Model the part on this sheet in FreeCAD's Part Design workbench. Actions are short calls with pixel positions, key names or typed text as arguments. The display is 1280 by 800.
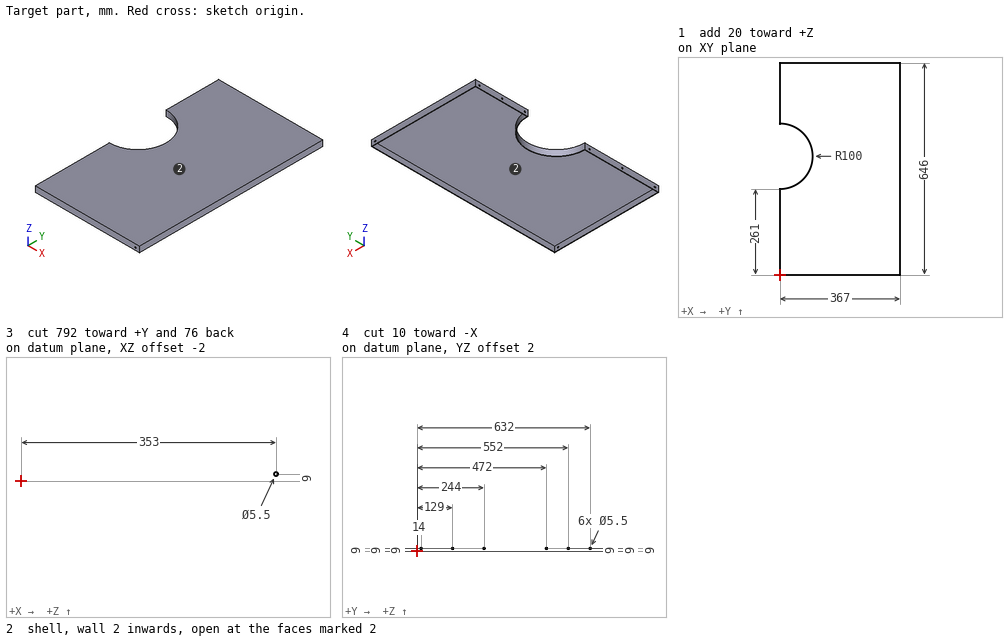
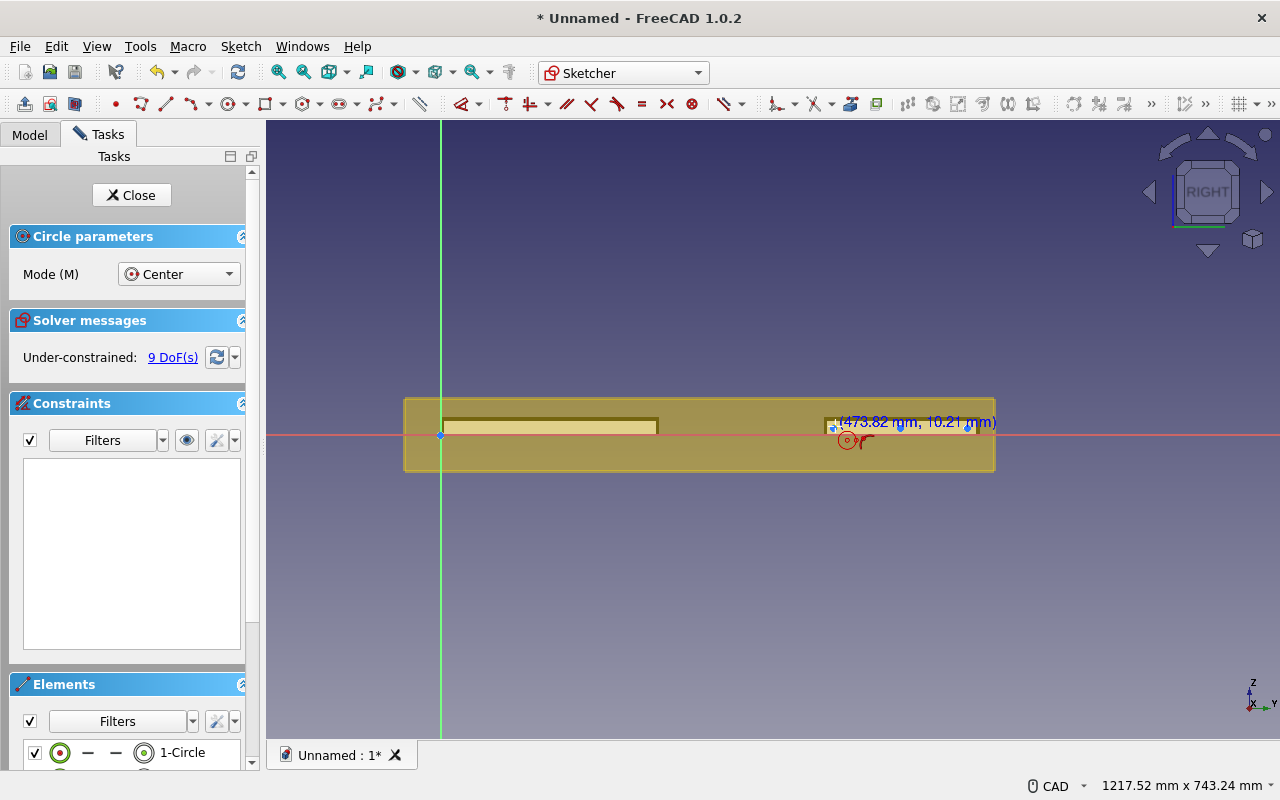
scroll(453, 428, up, 12)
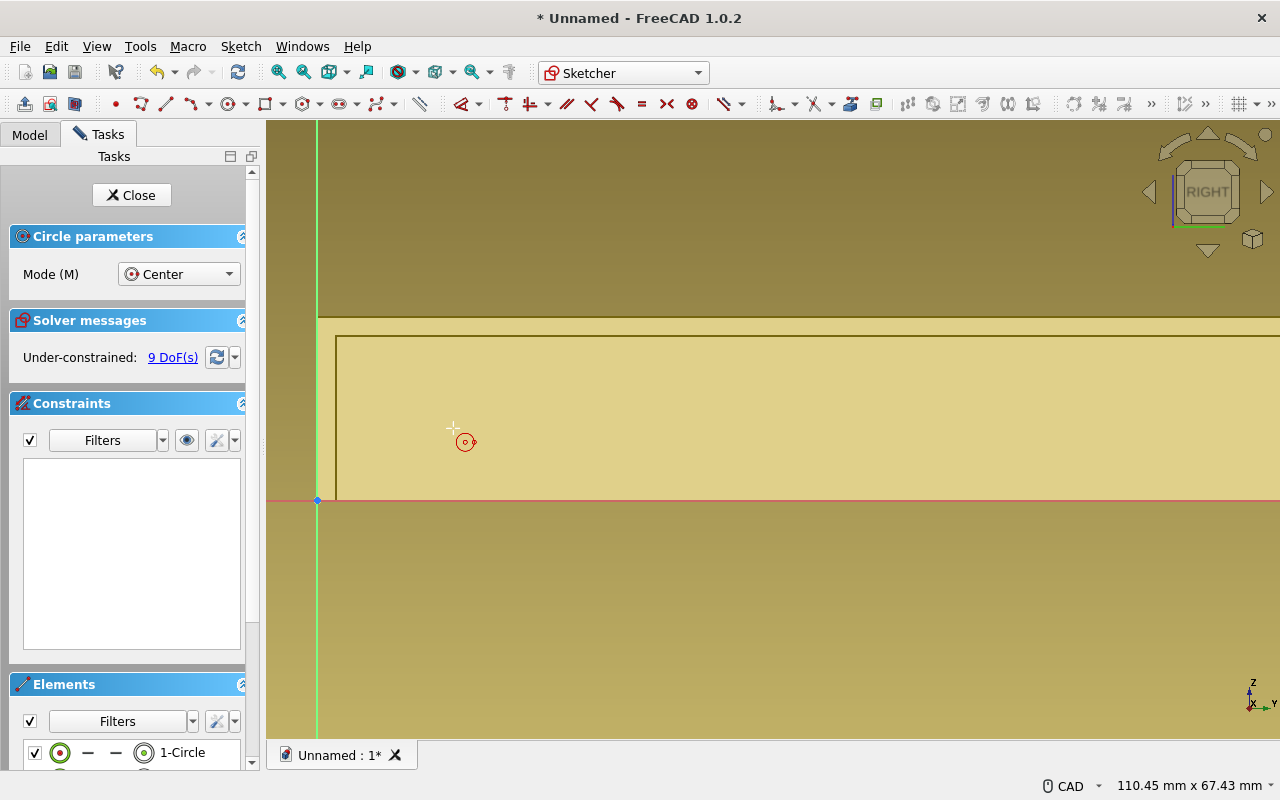
scroll(452, 428, down, 12)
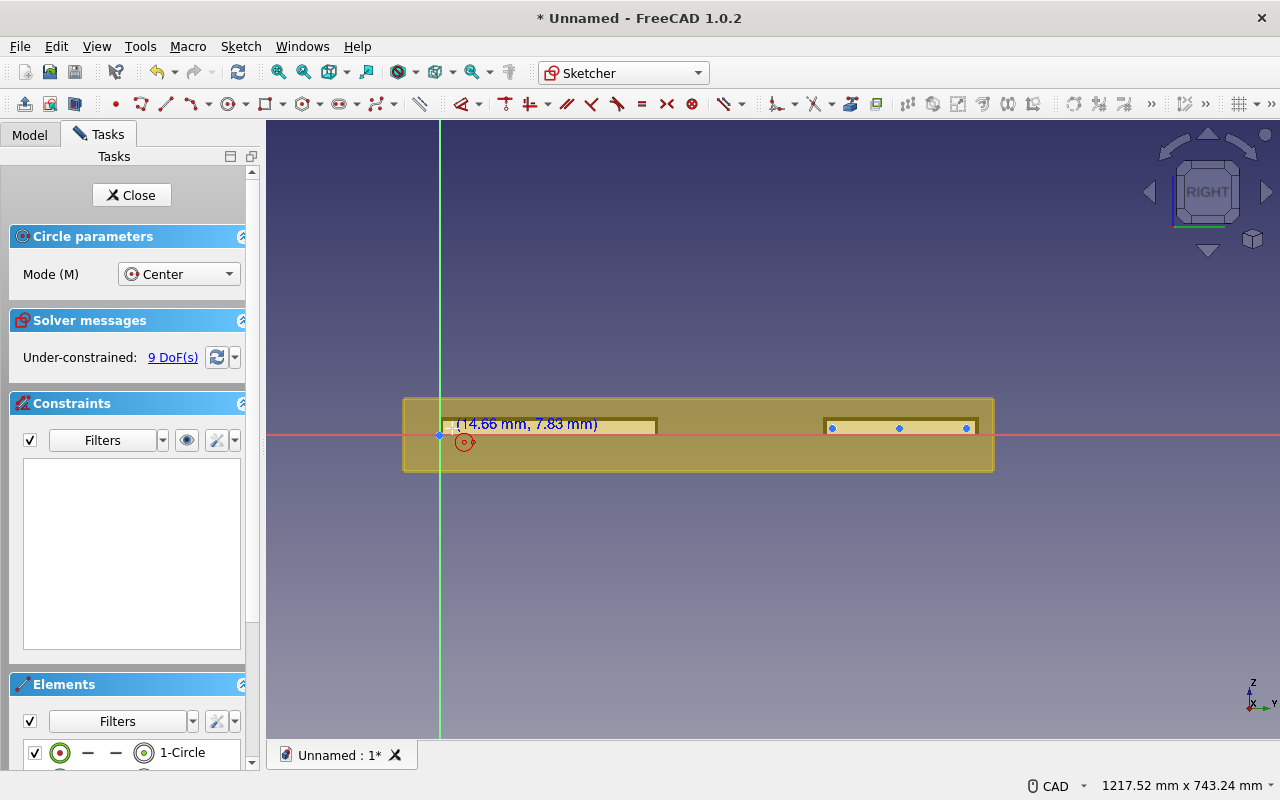
scroll(452, 428, up, 4)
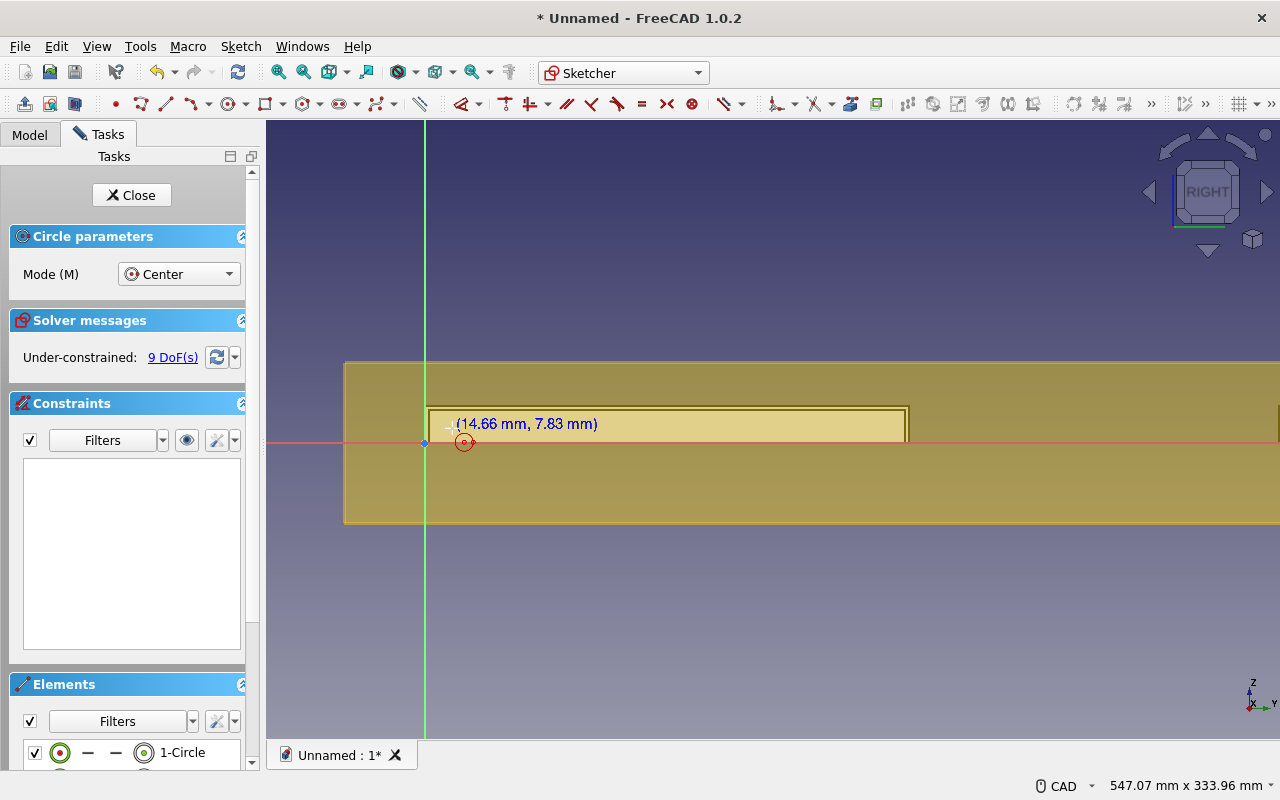
click(451, 426)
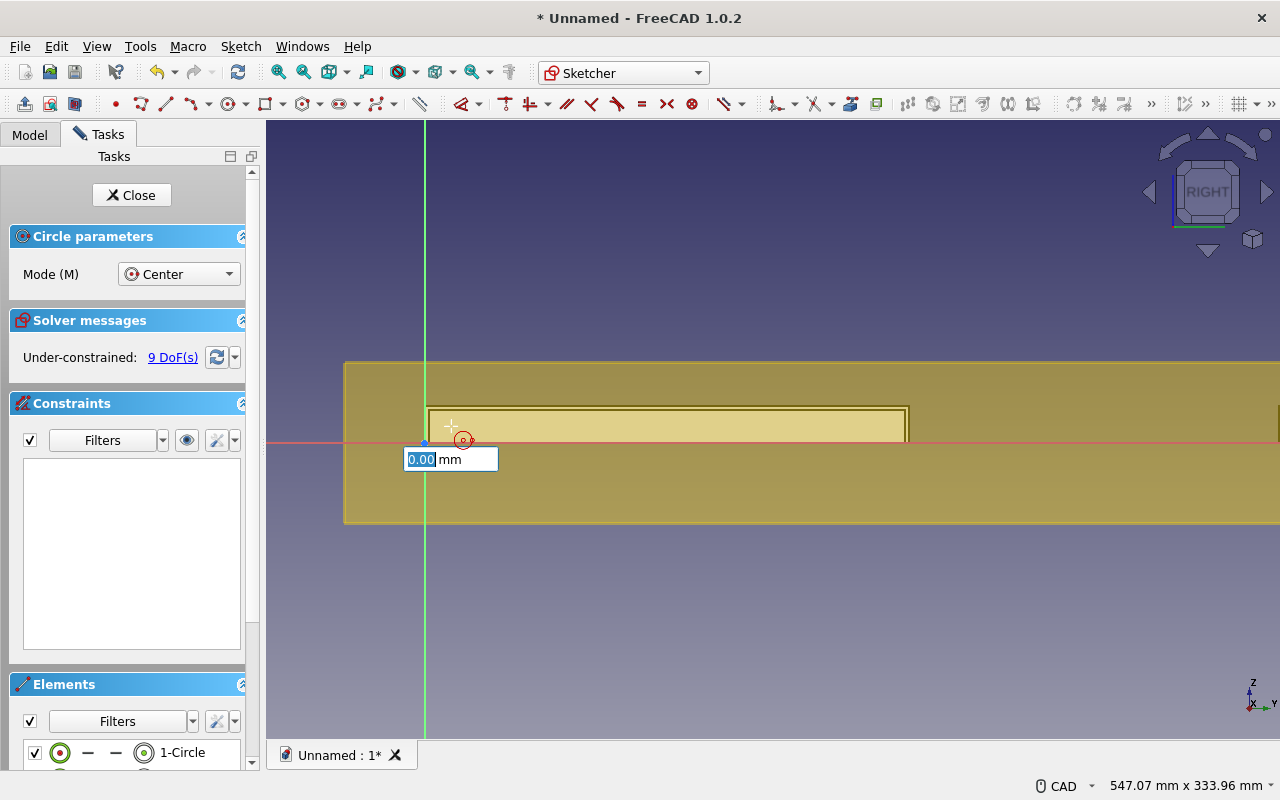
scroll(455, 423, up, 6)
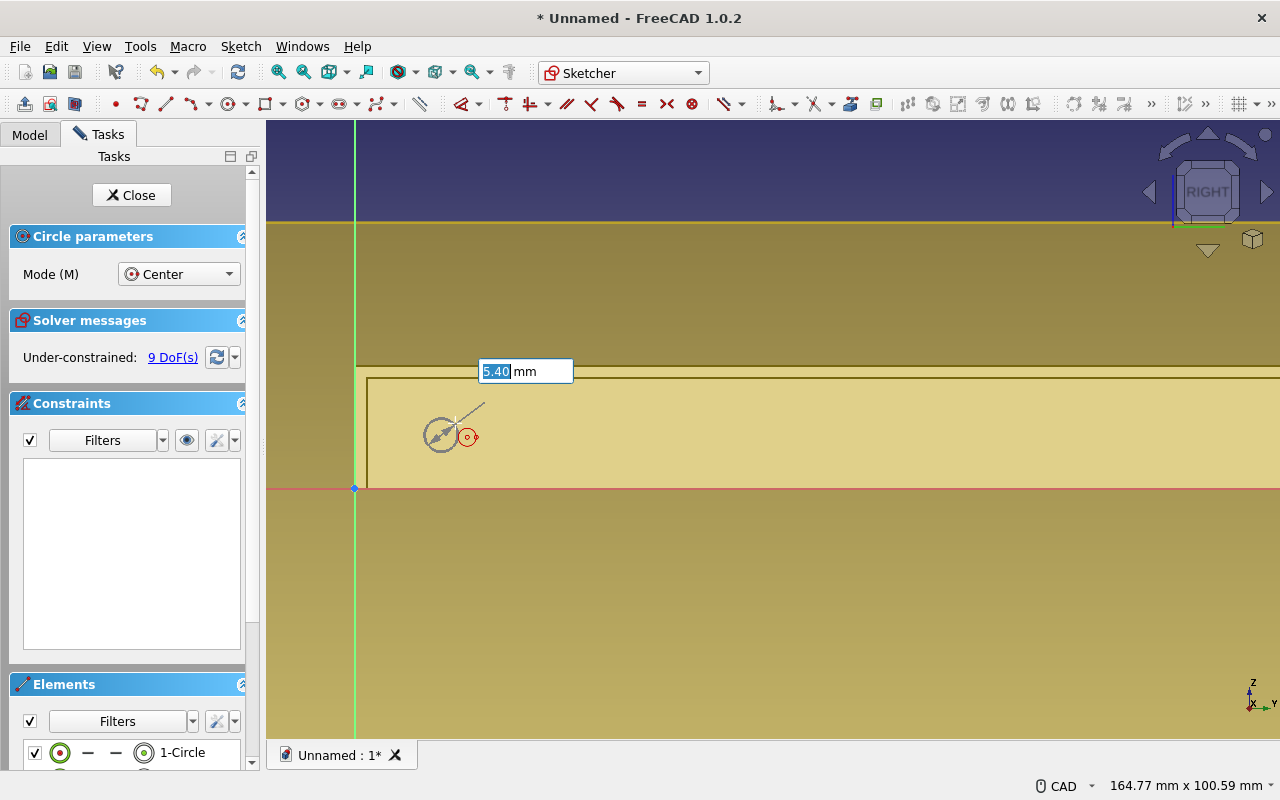
click(453, 421)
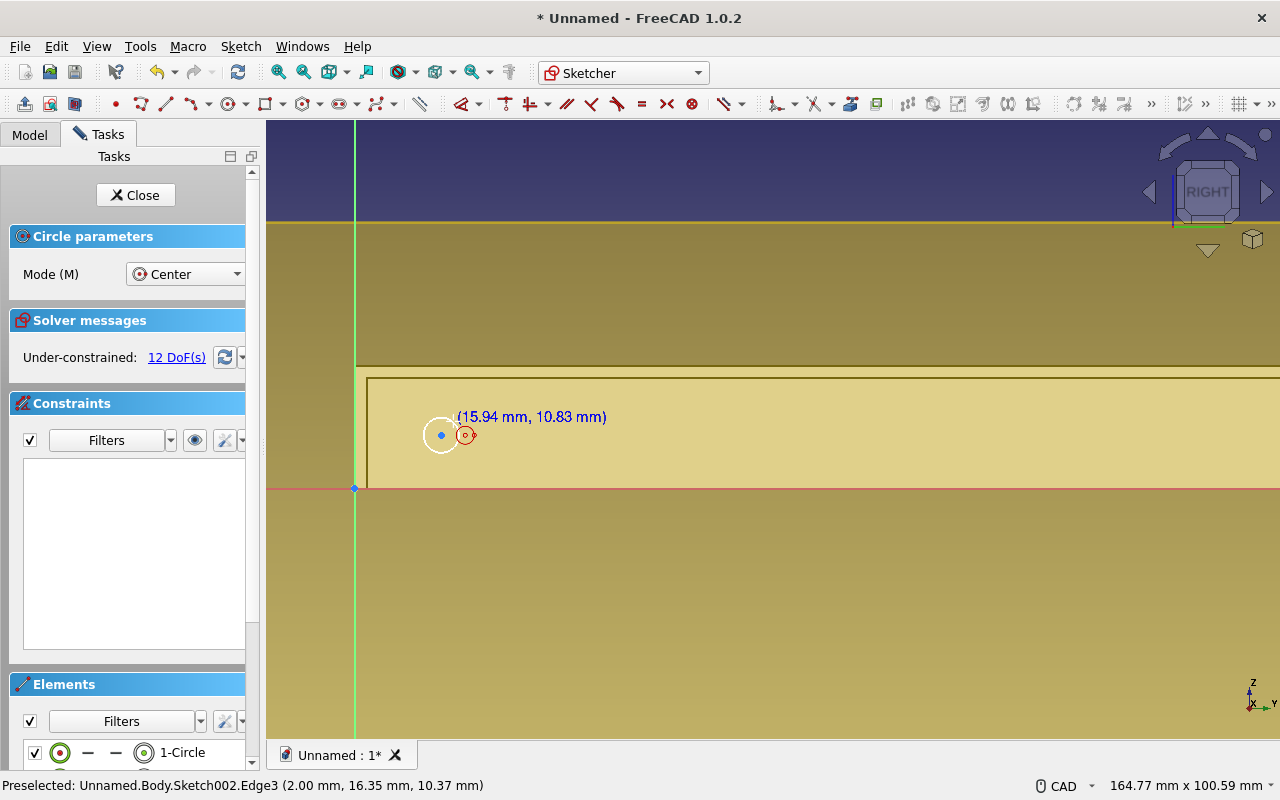
scroll(454, 426, down, 10)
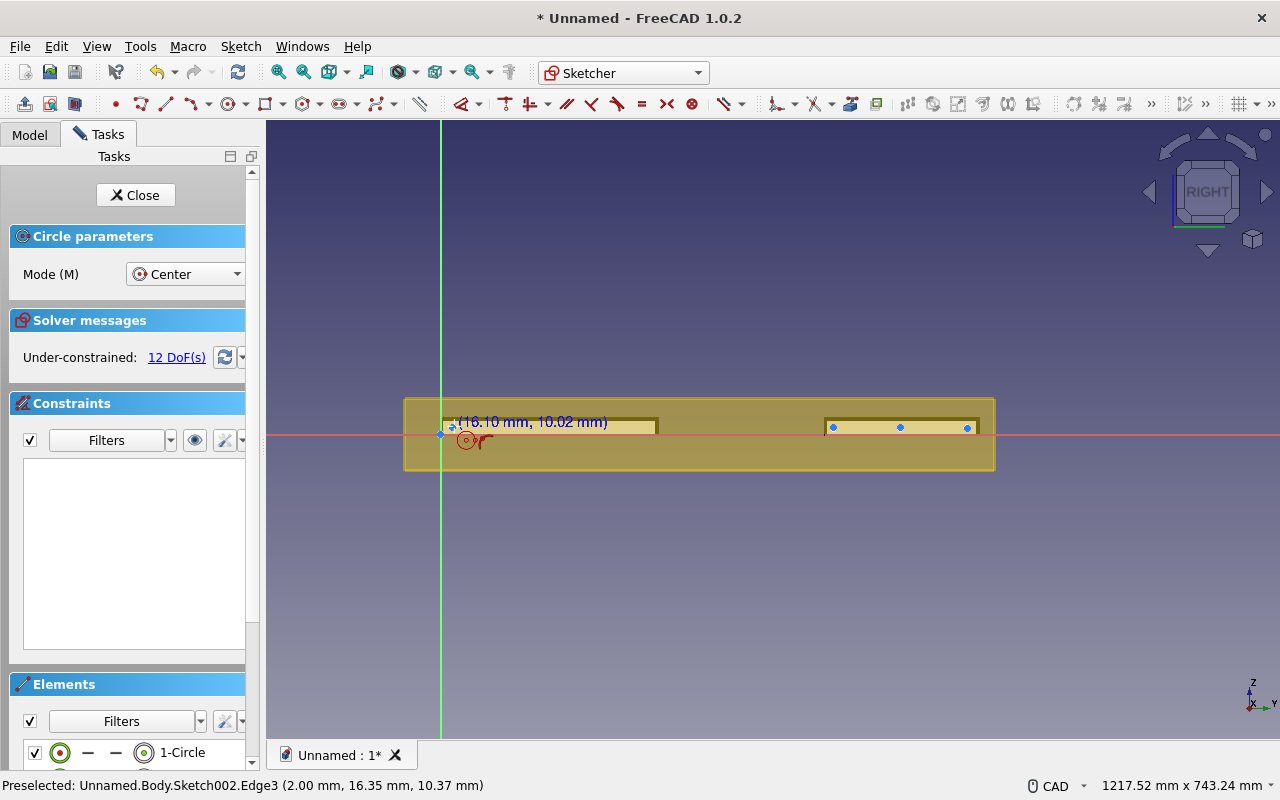
scroll(548, 427, up, 12)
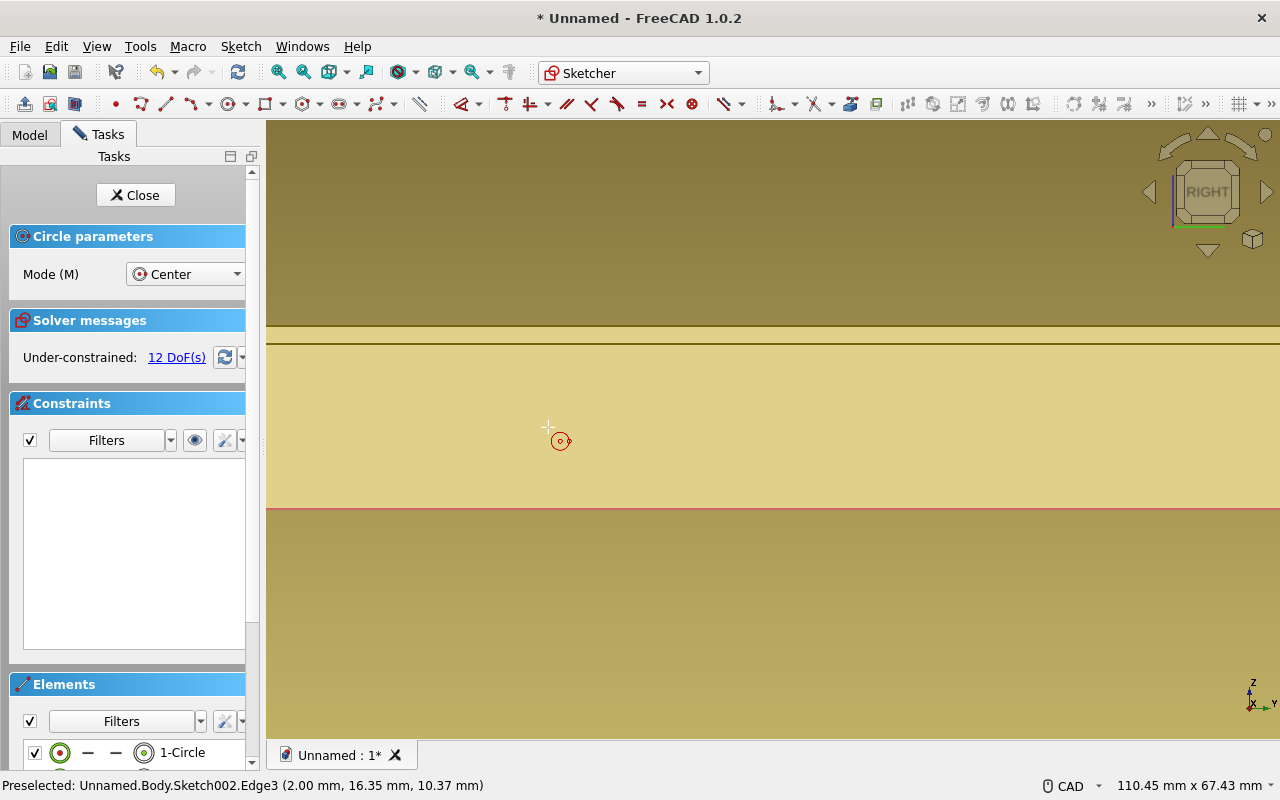
scroll(548, 427, down, 12)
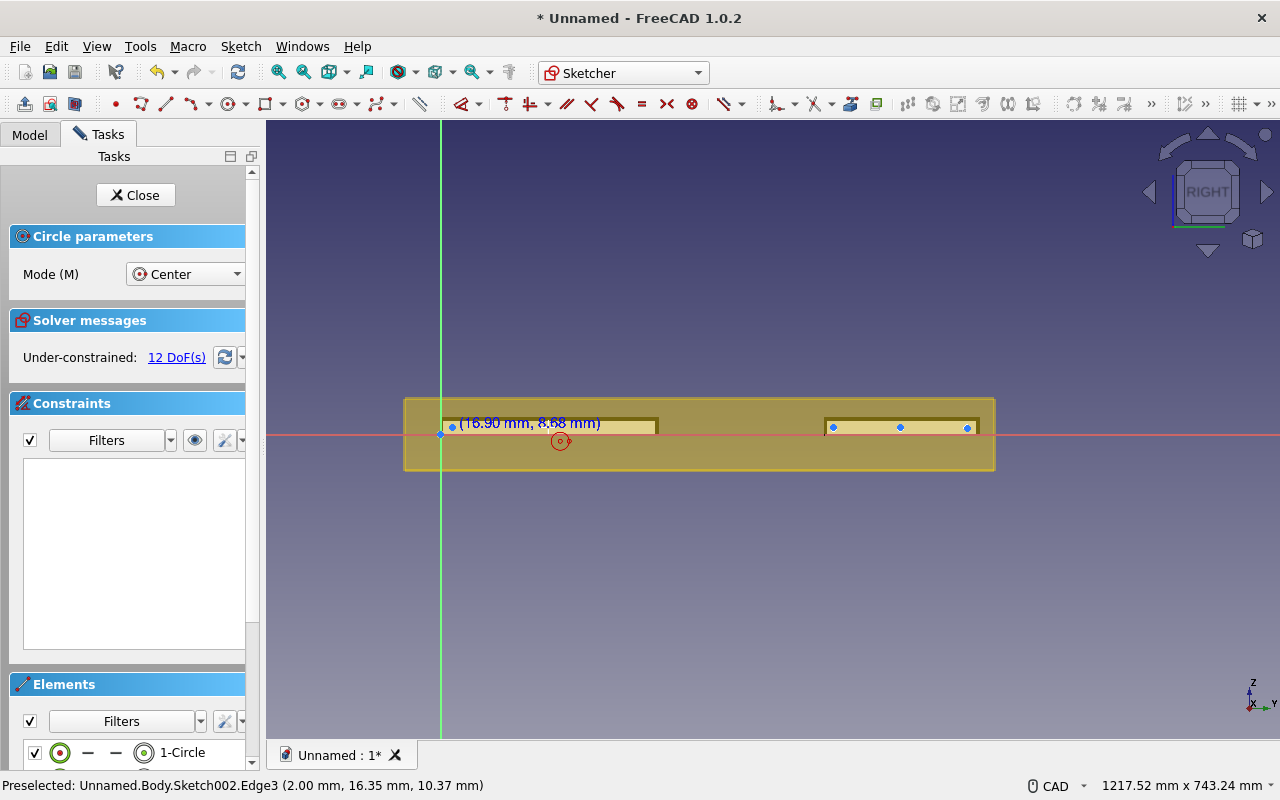
scroll(548, 427, up, 4)